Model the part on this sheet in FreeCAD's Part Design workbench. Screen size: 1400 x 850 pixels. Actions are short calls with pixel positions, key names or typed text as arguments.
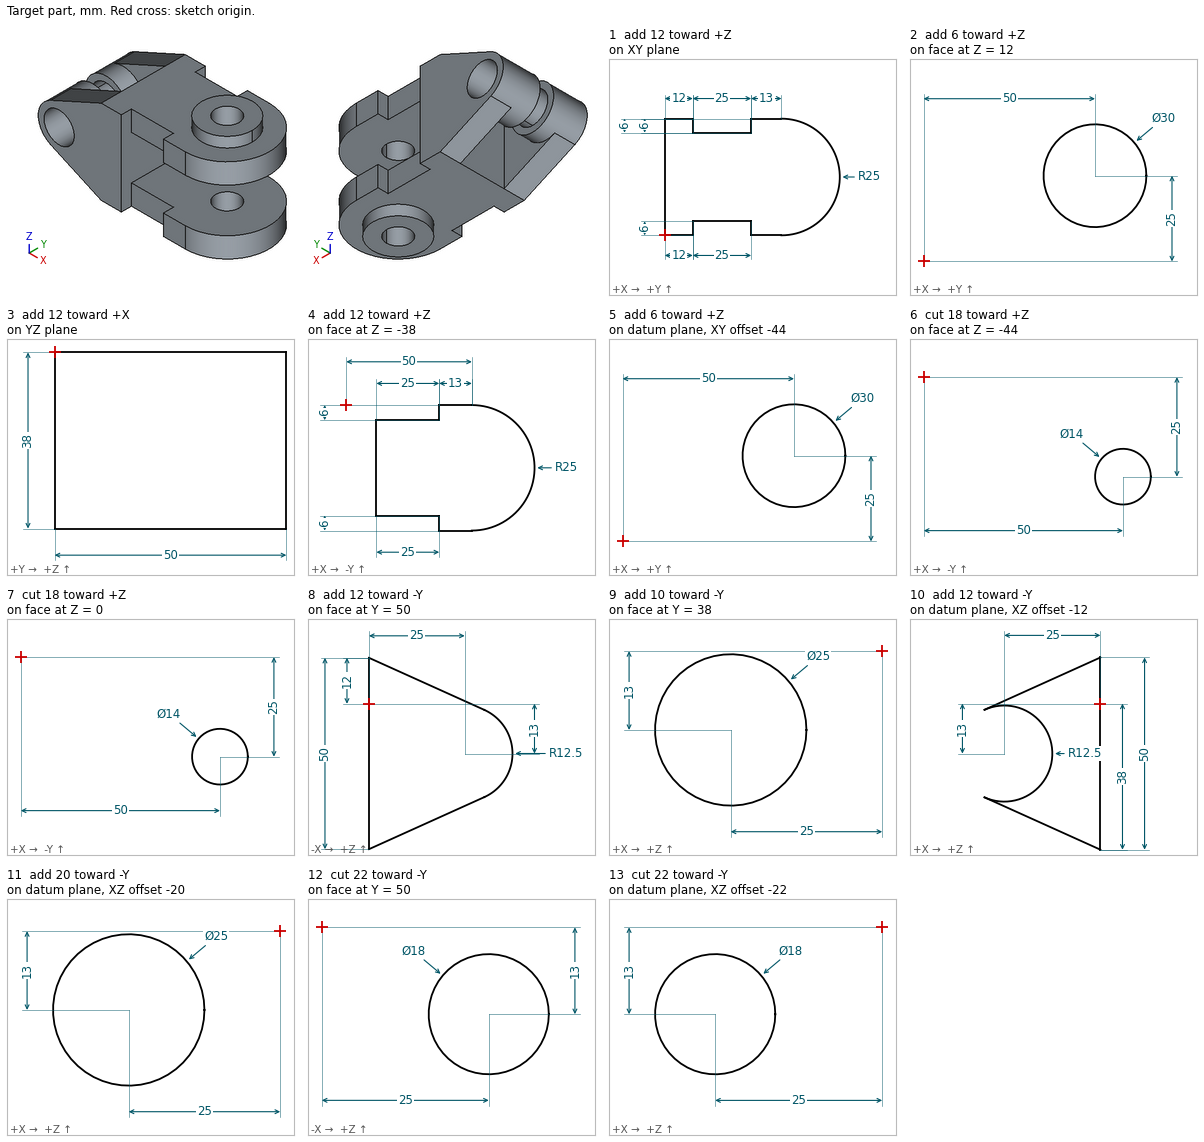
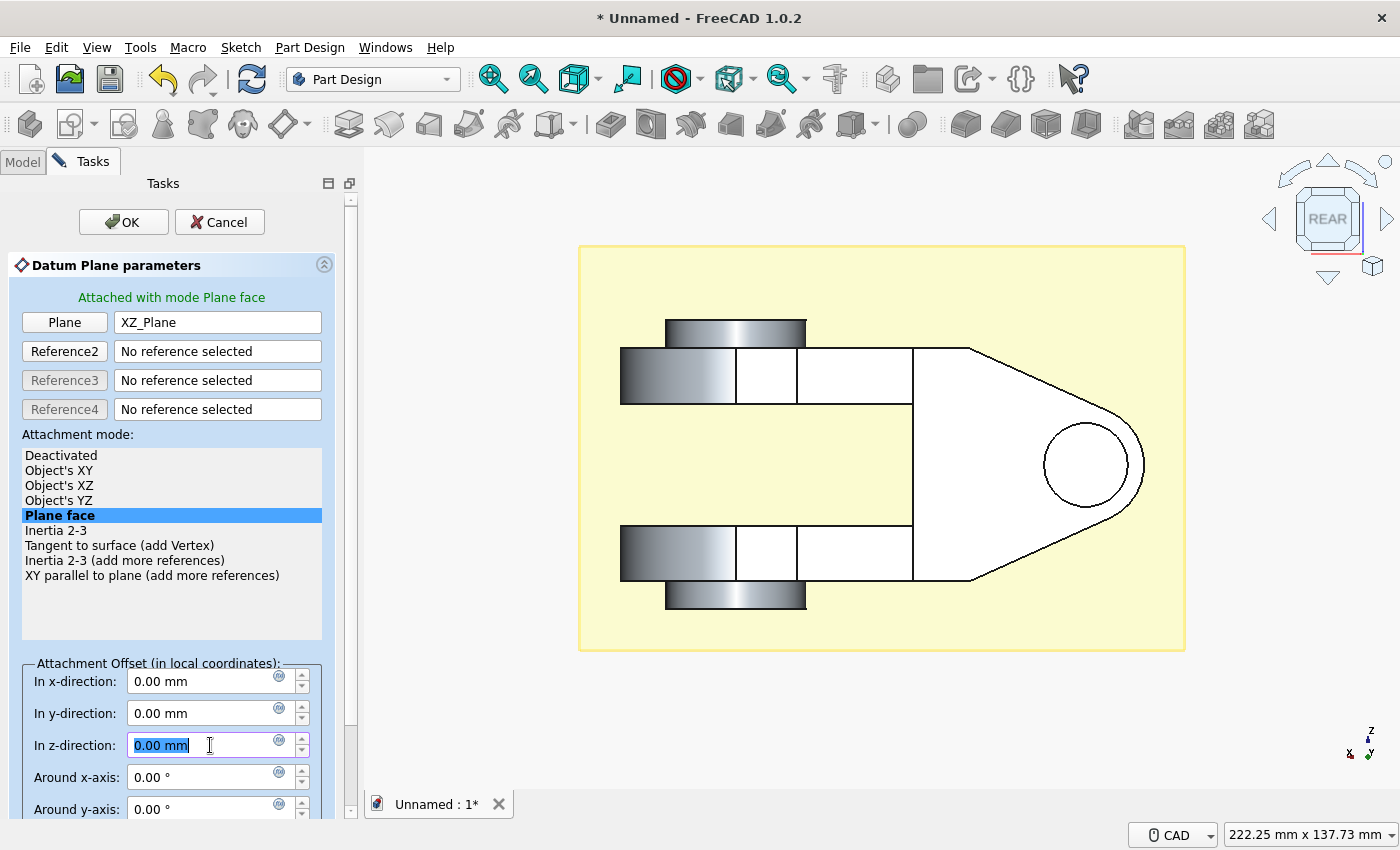
text(-22)
key(Tab)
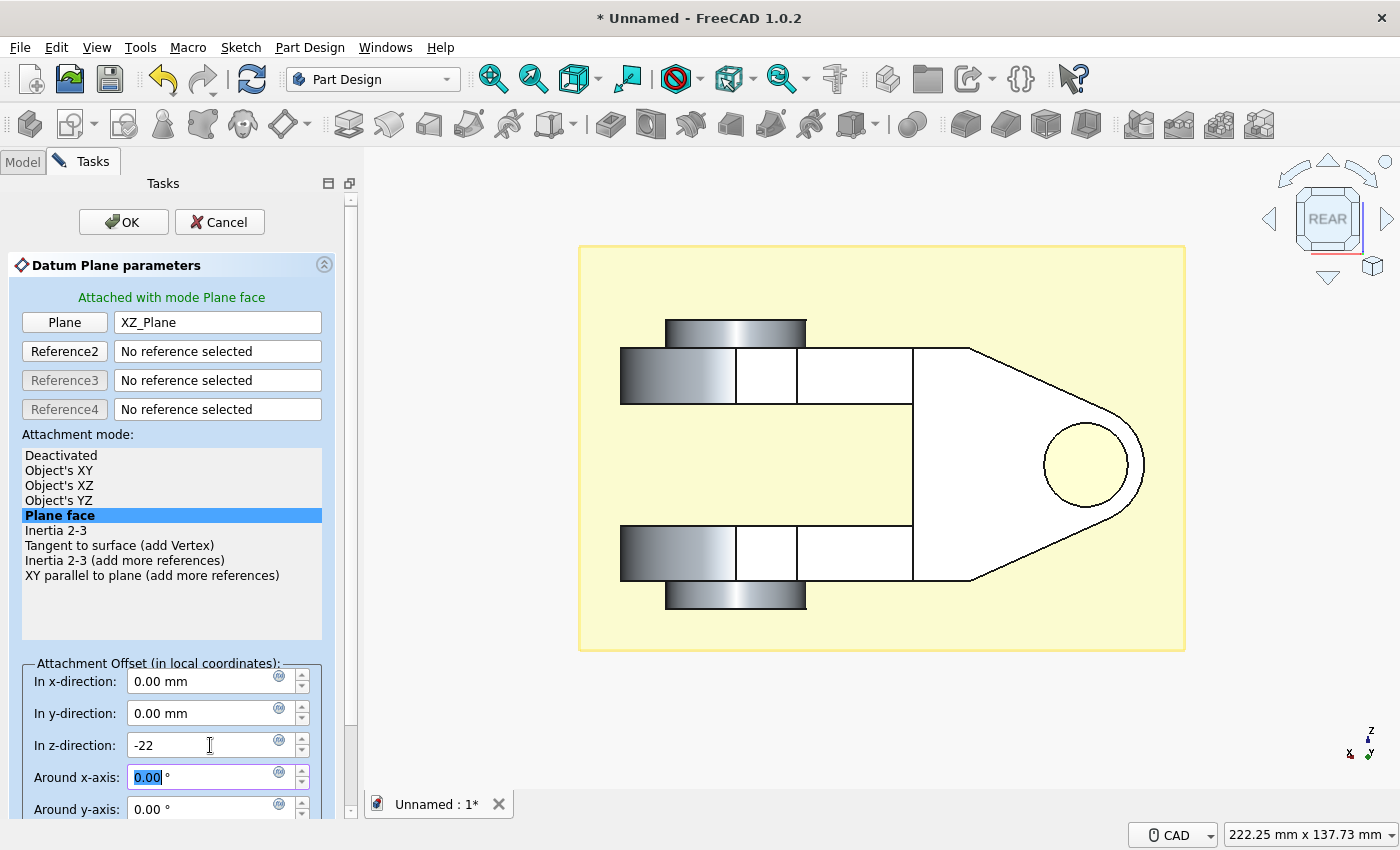
click(124, 222)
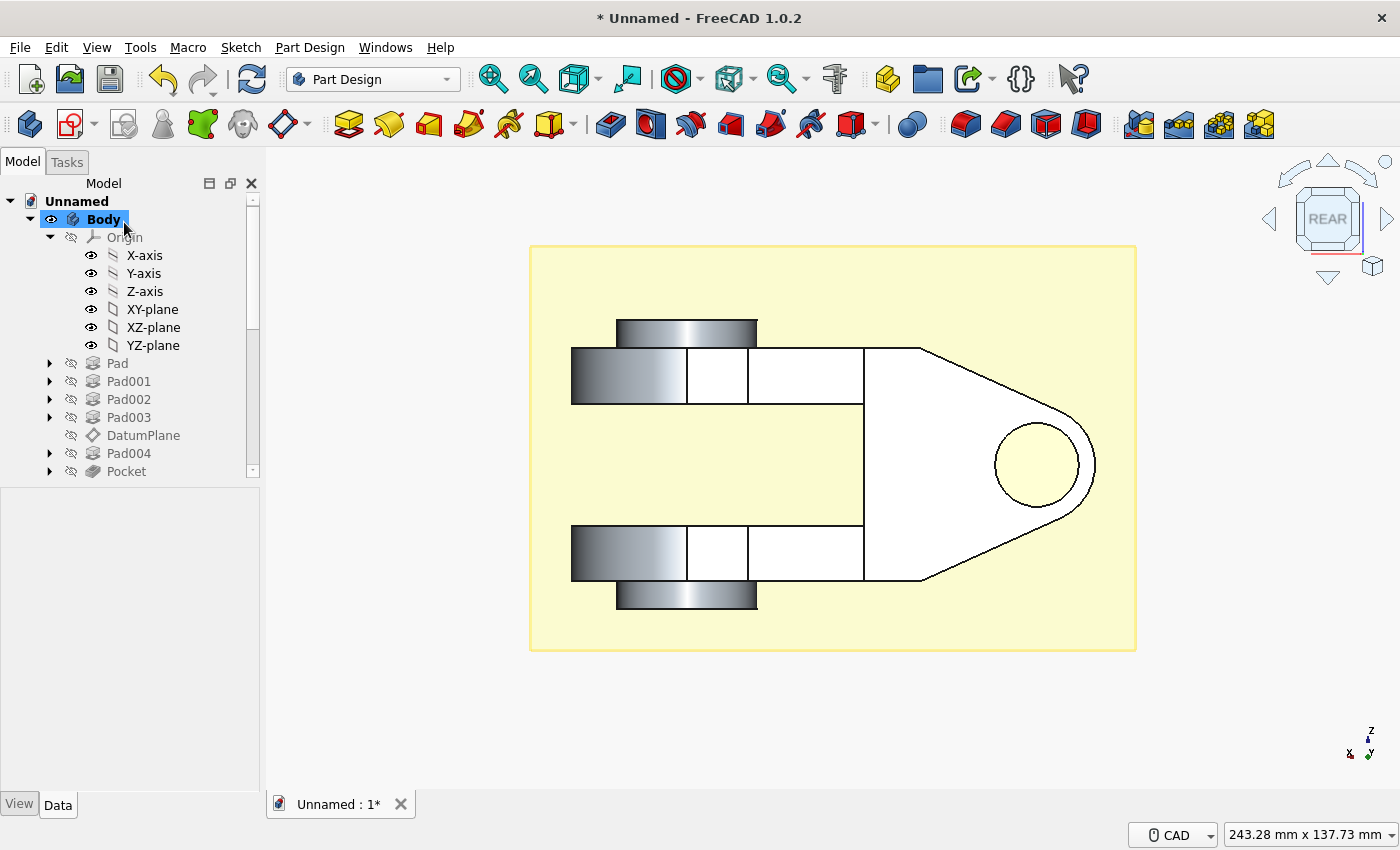
scroll(100, 341, down, 3)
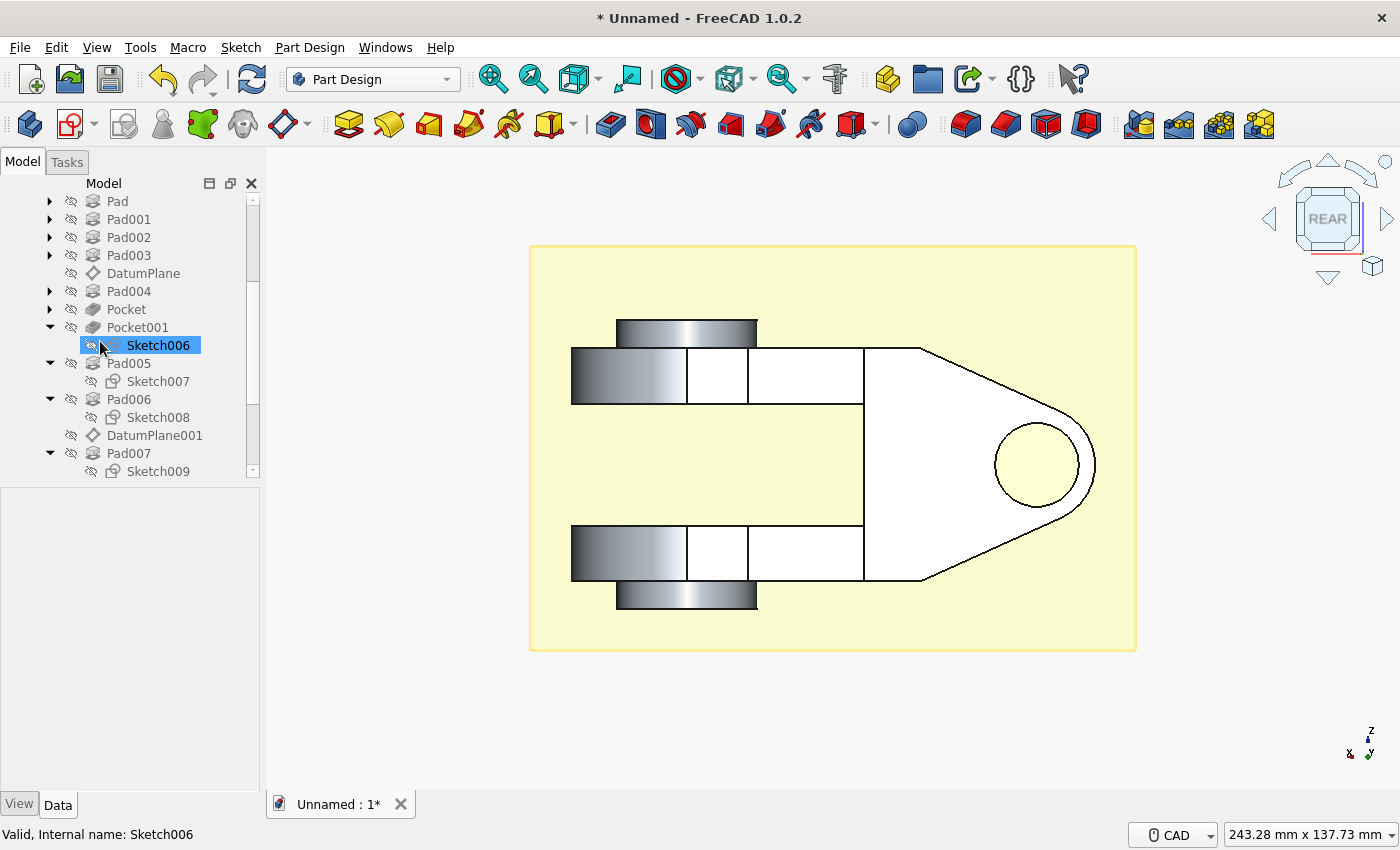
scroll(140, 341, up, 15)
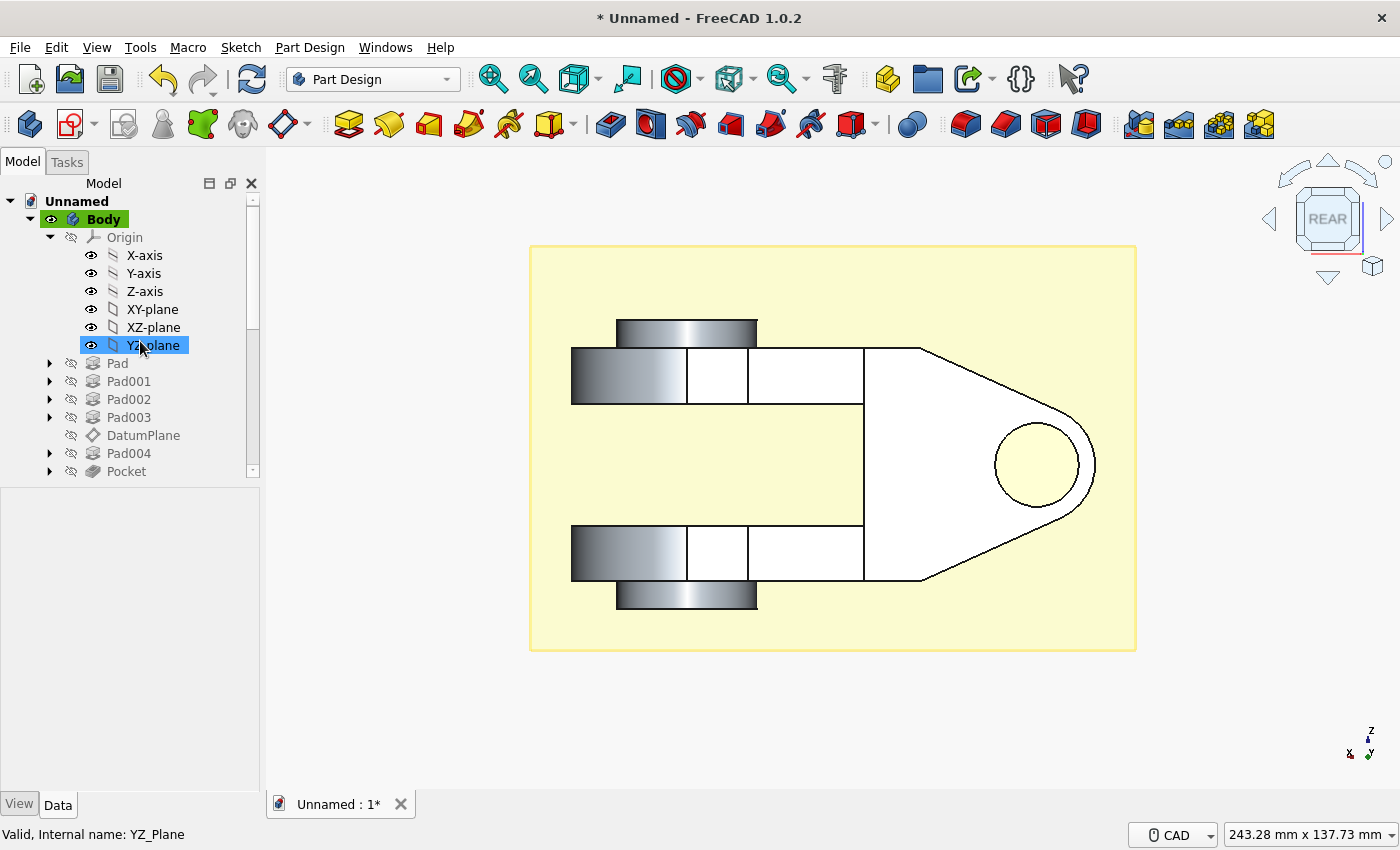
scroll(100, 341, down, 6)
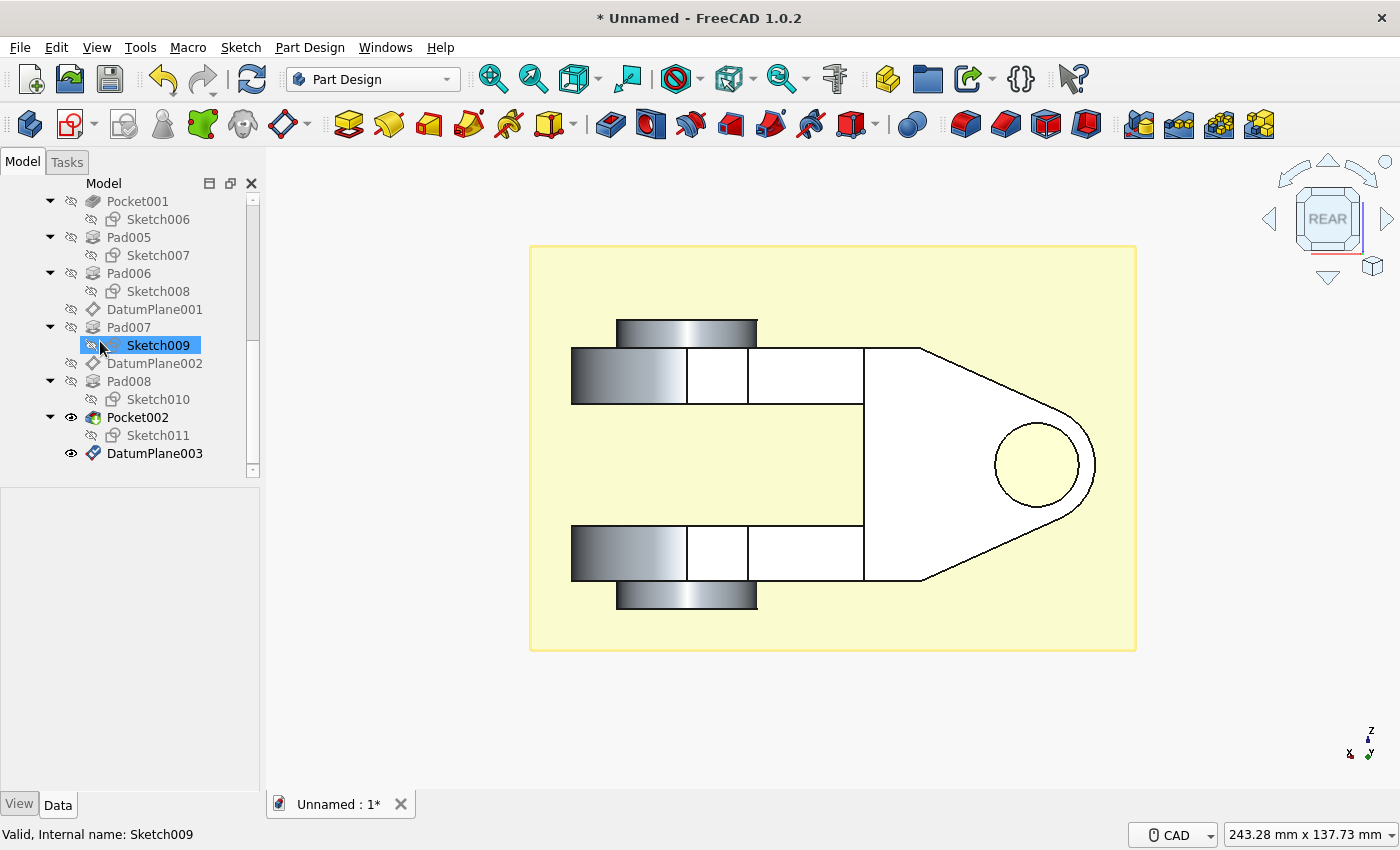
click(116, 453)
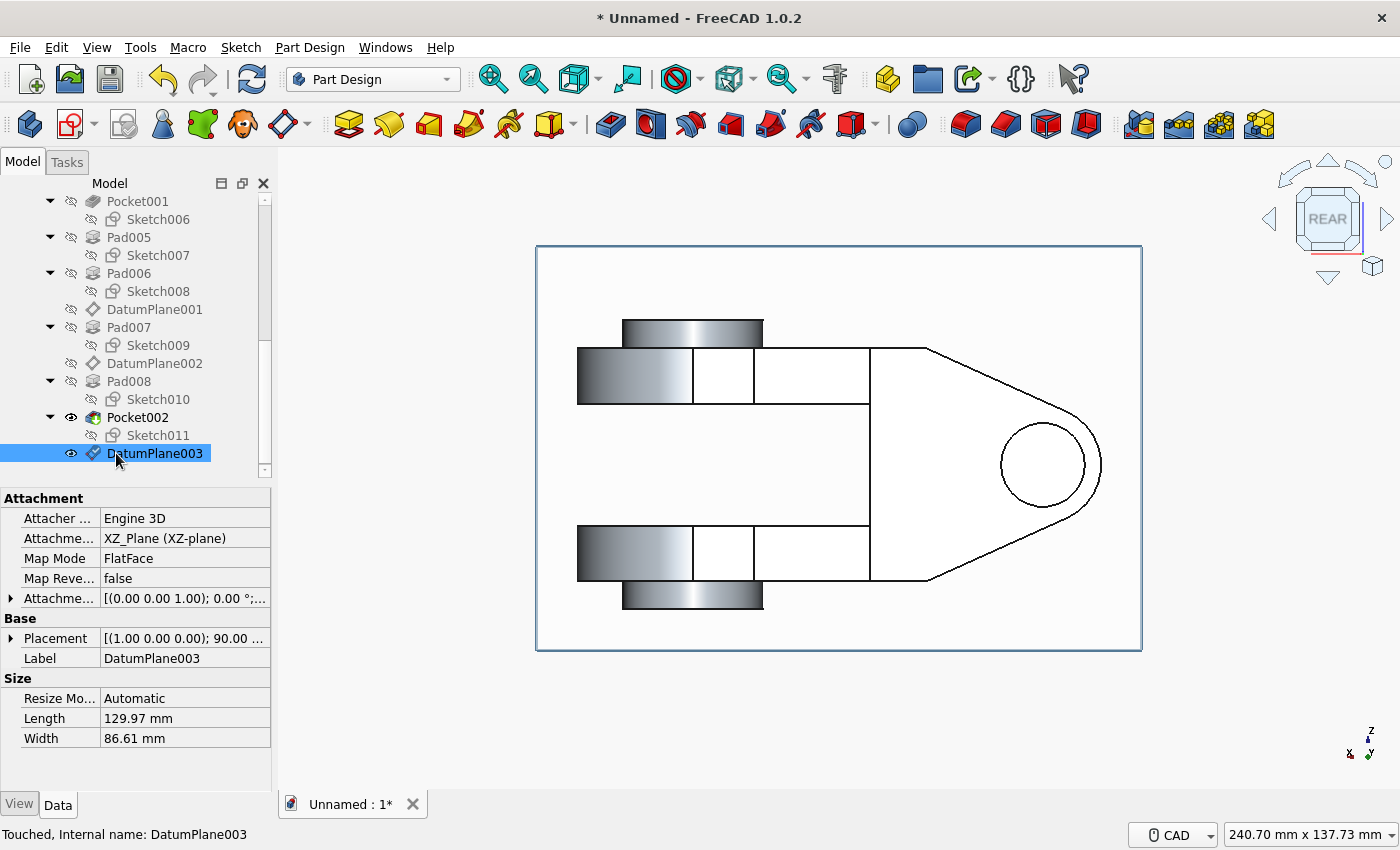
click(70, 124)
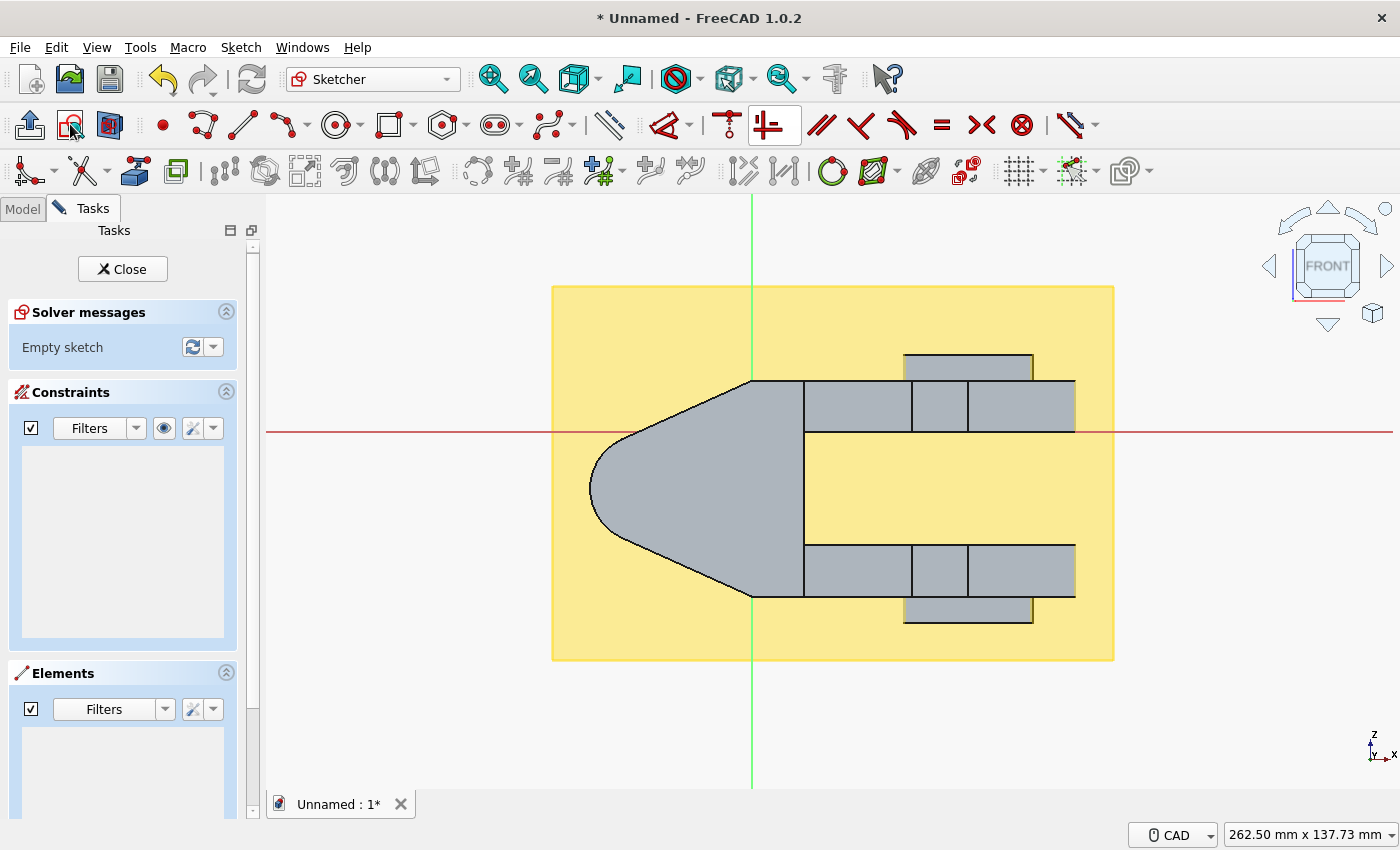
click(110, 126)